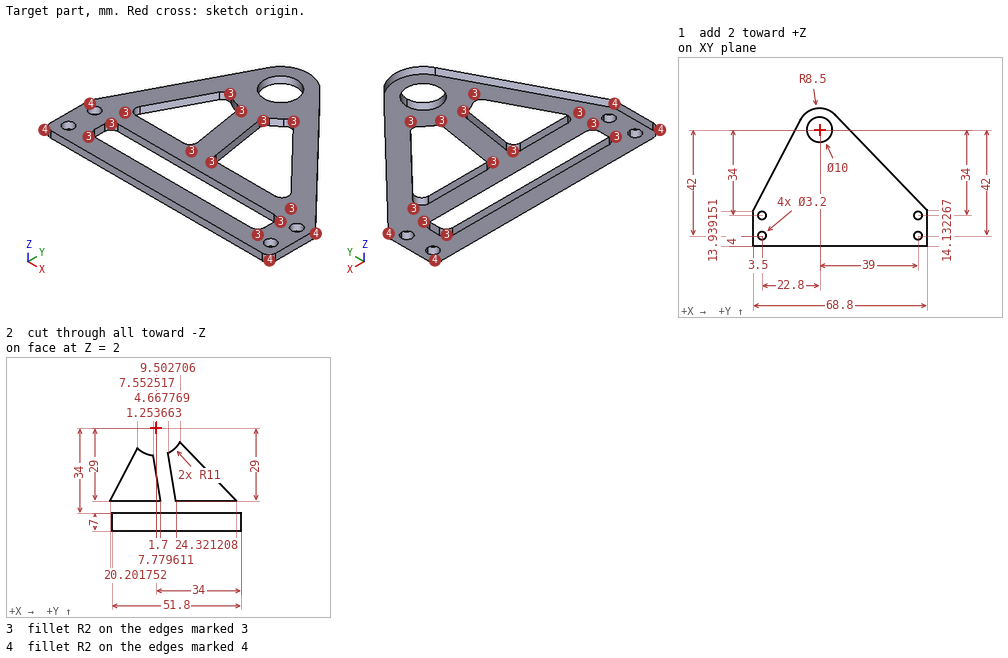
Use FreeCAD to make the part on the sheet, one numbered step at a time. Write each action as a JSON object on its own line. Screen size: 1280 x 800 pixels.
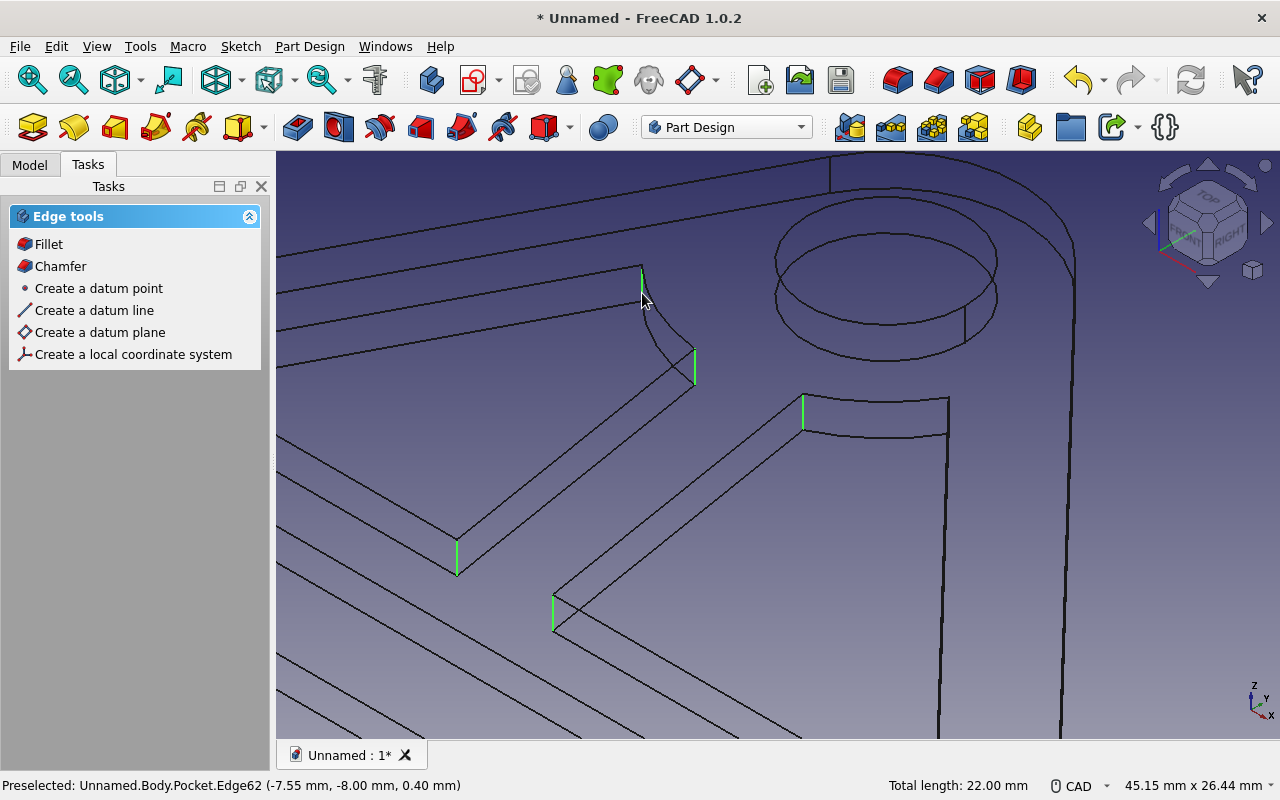
{"action": "left_click", "coordinate": [33, 80]}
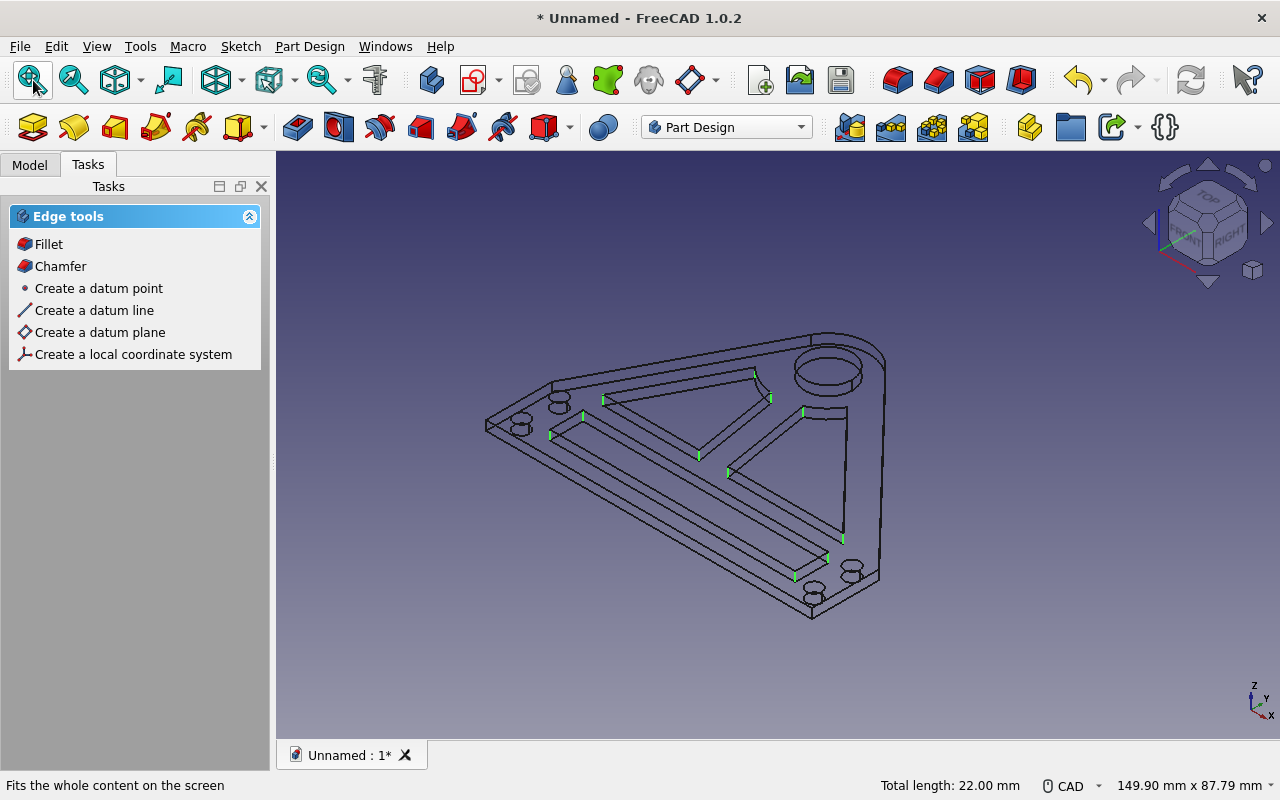
{"action": "key", "text": "2"}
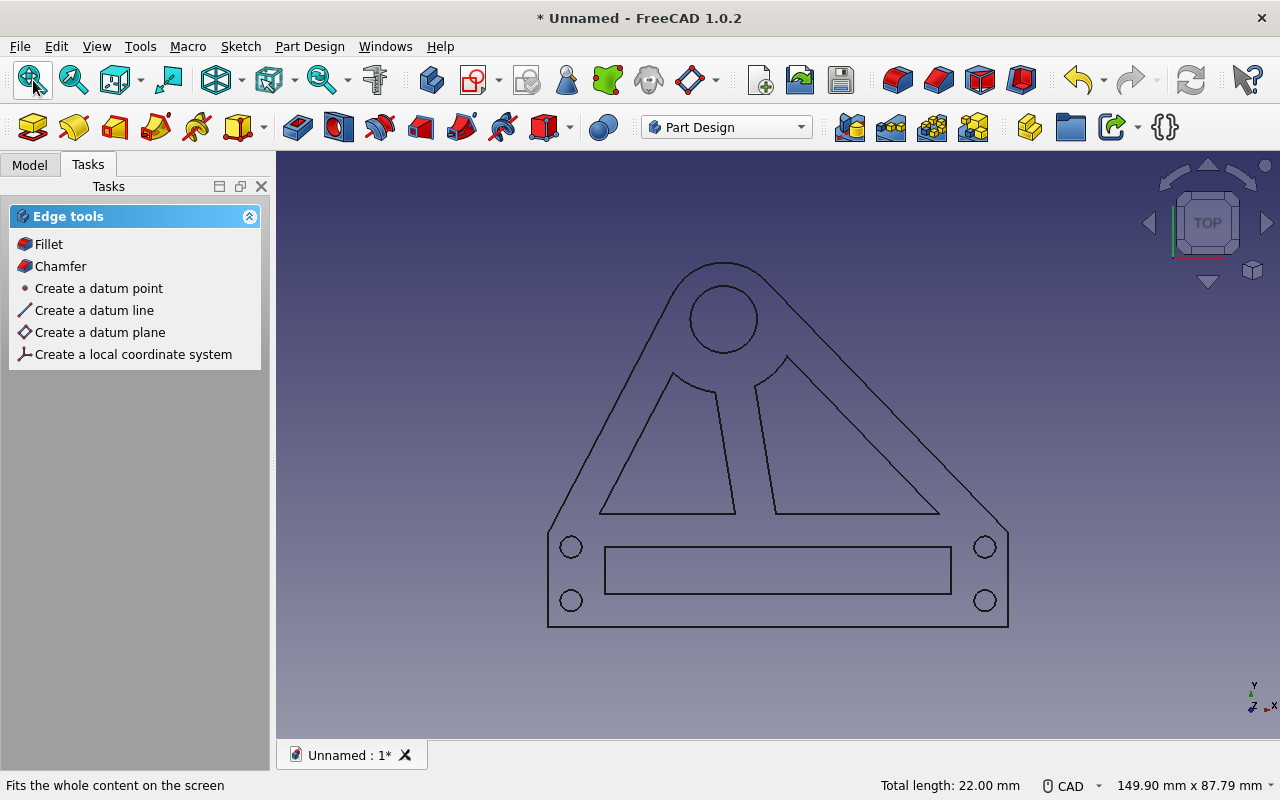
{"action": "scroll", "coordinate": [787, 355], "scroll_direction": "up", "scroll_amount": 6}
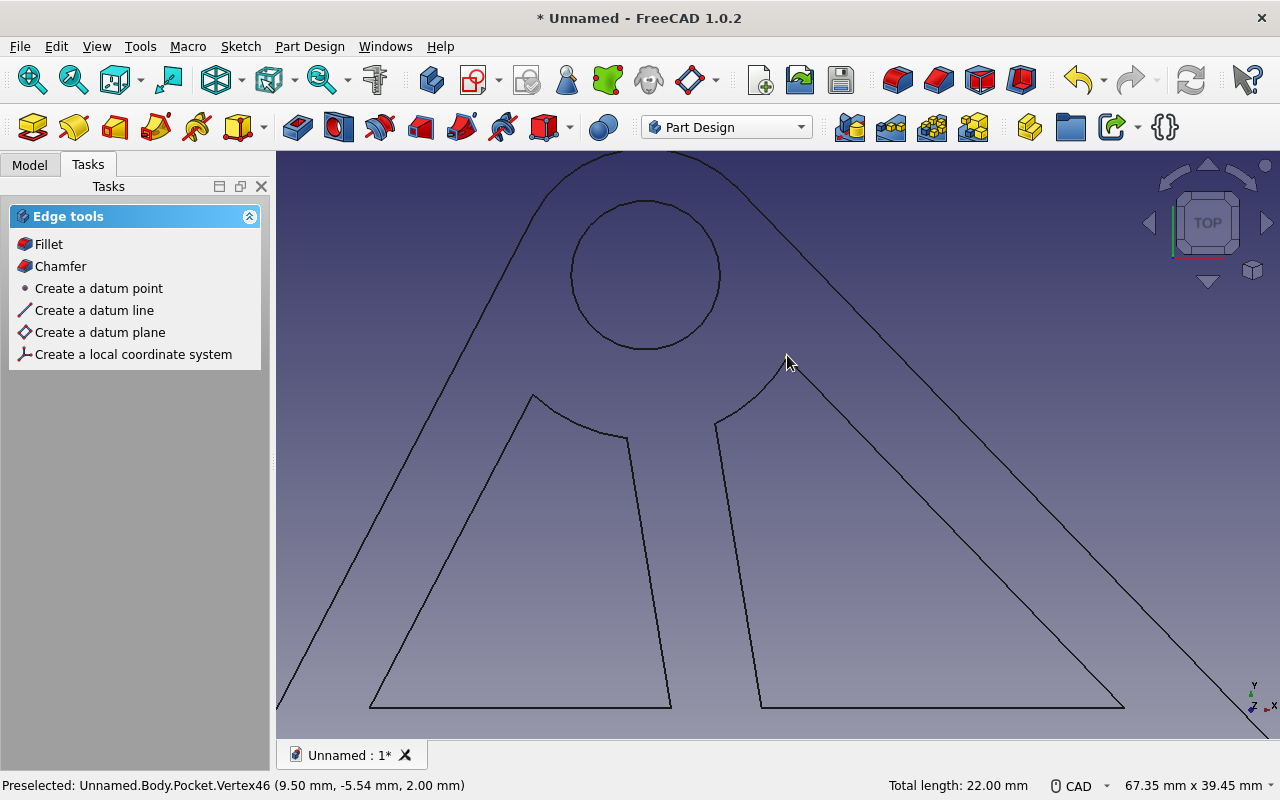
{"action": "left_click", "coordinate": [33, 80]}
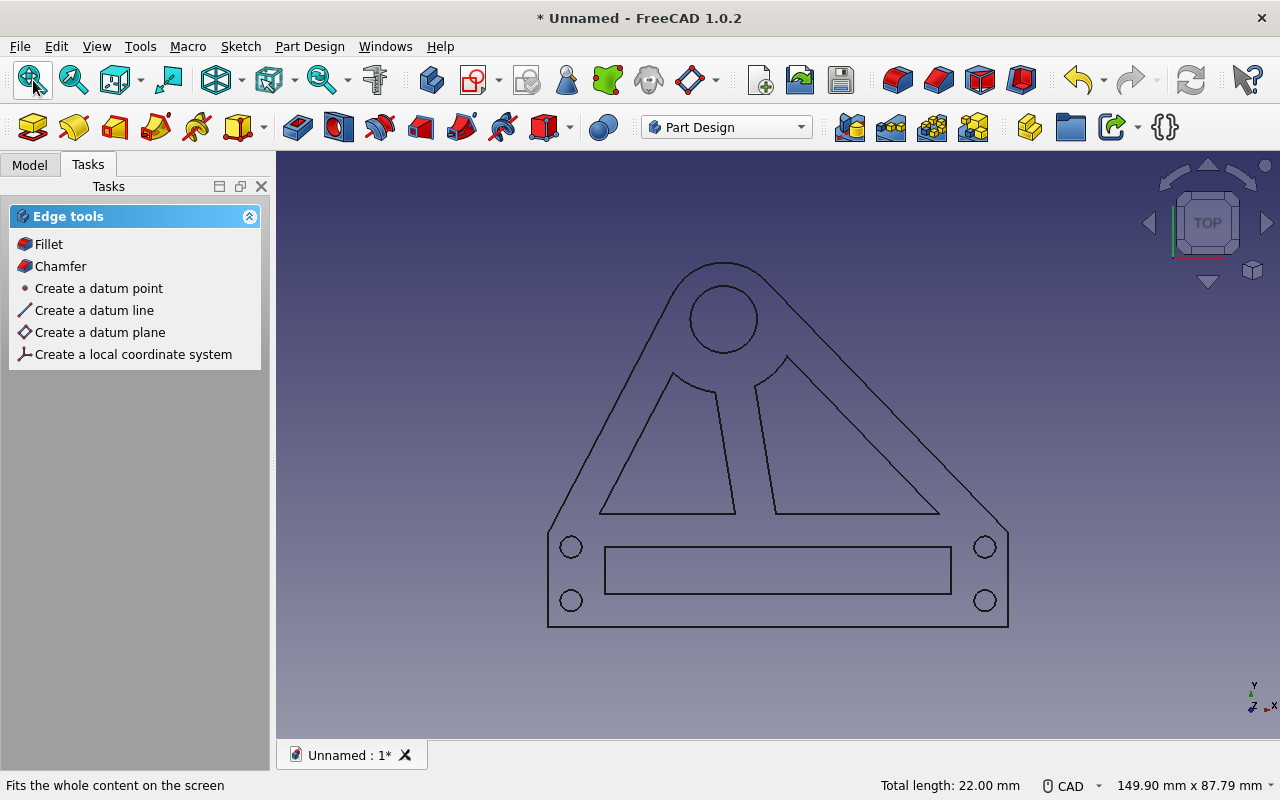
{"action": "key", "text": "1"}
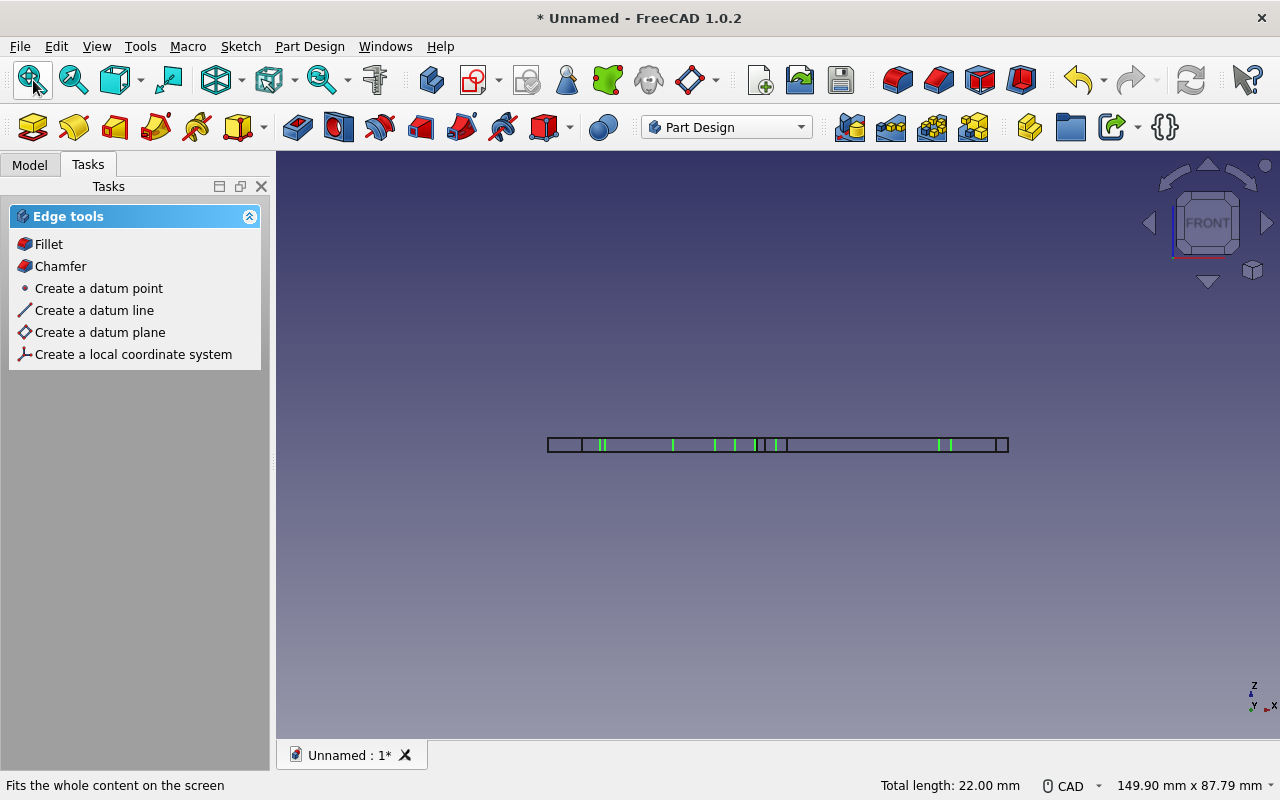
{"action": "left_click", "coordinate": [787, 444], "text": "ctrl"}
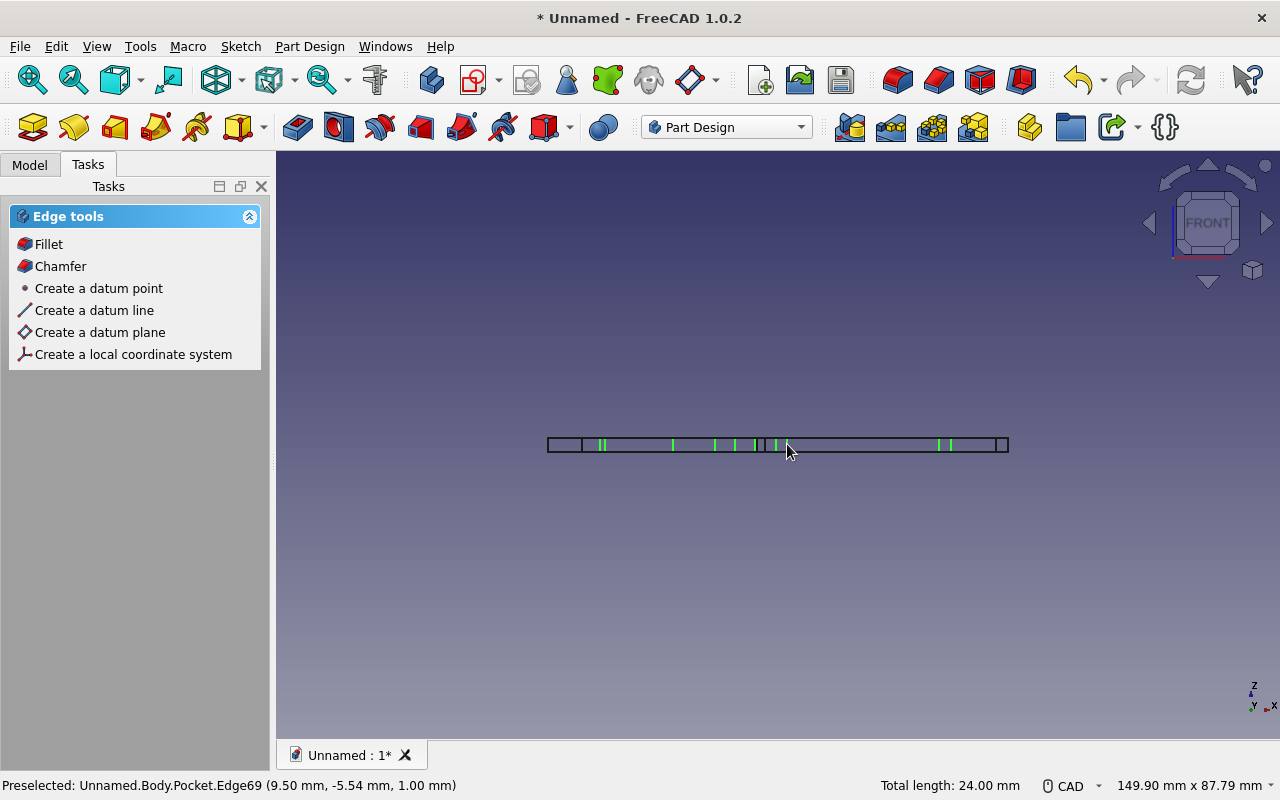
{"action": "key", "text": "v 1"}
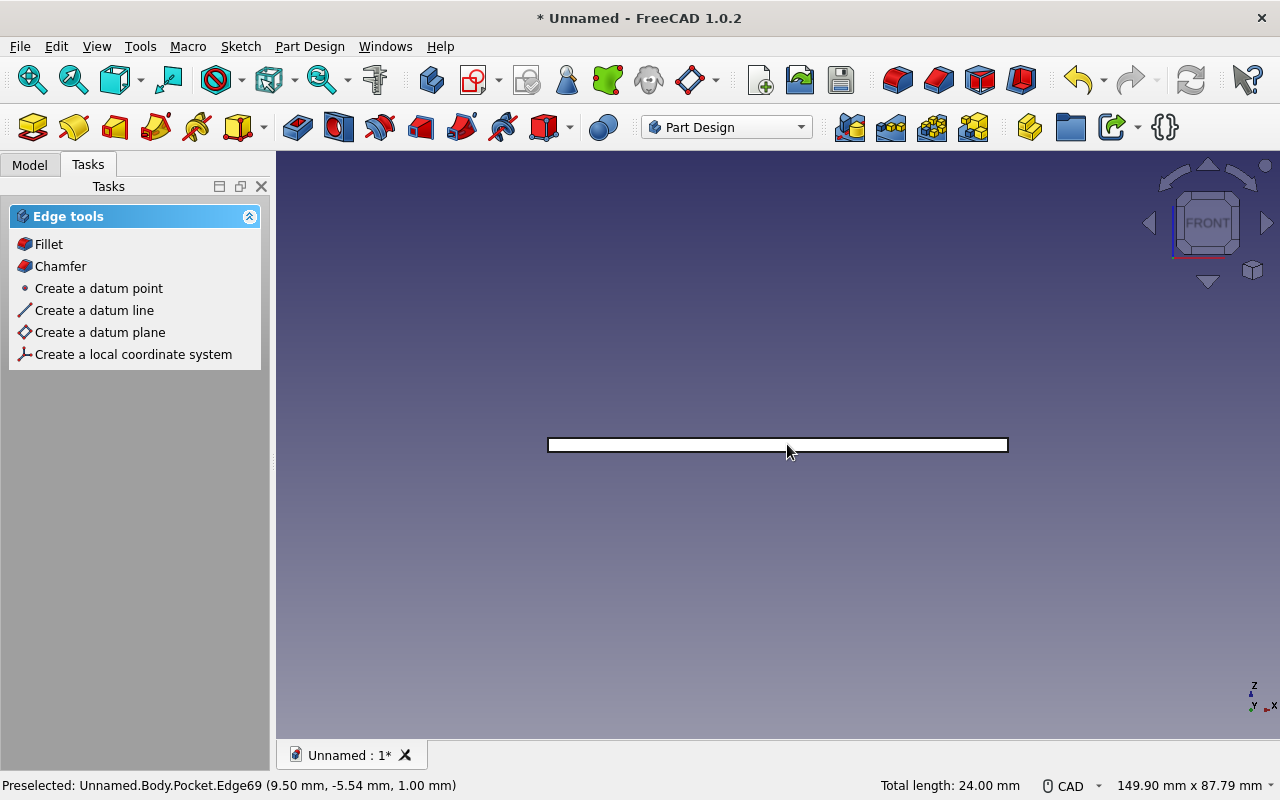
{"action": "left_click", "coordinate": [898, 80]}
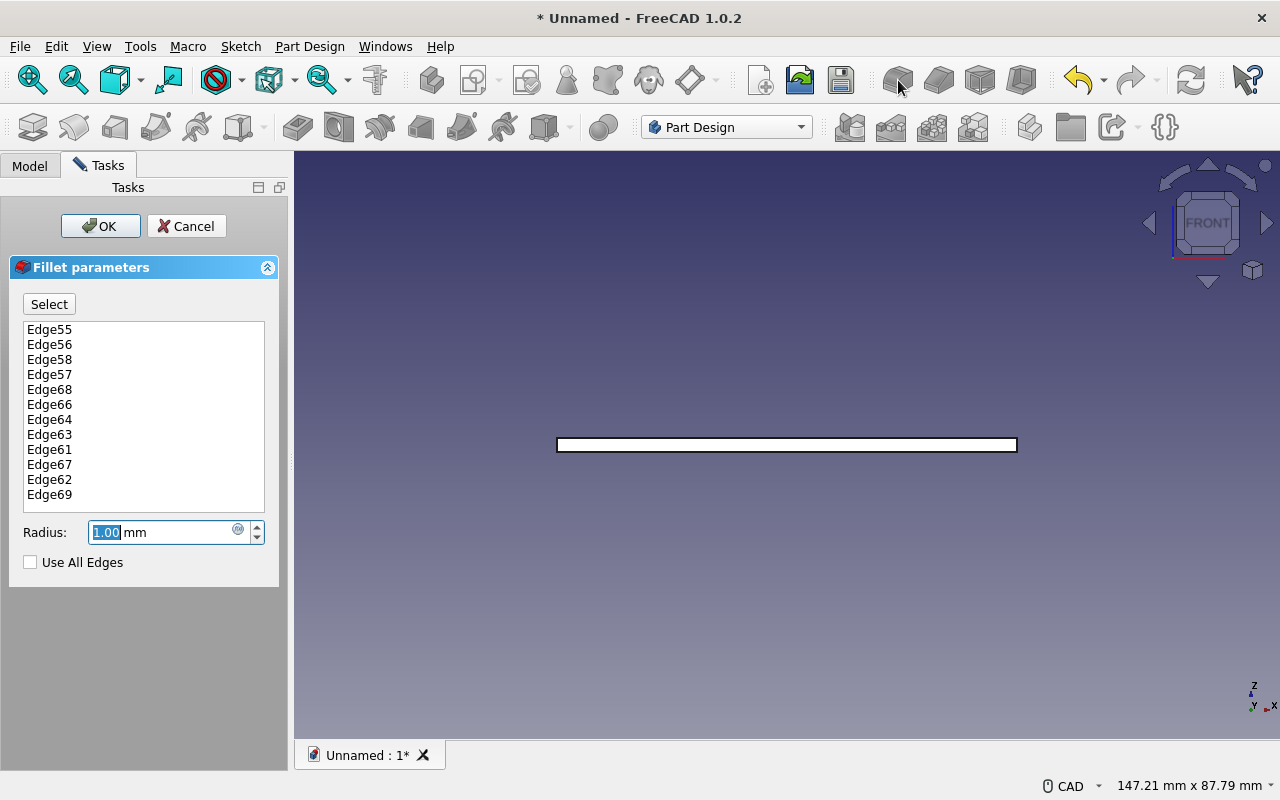
{"action": "type", "text": "2"}
{"action": "key", "text": "Tab"}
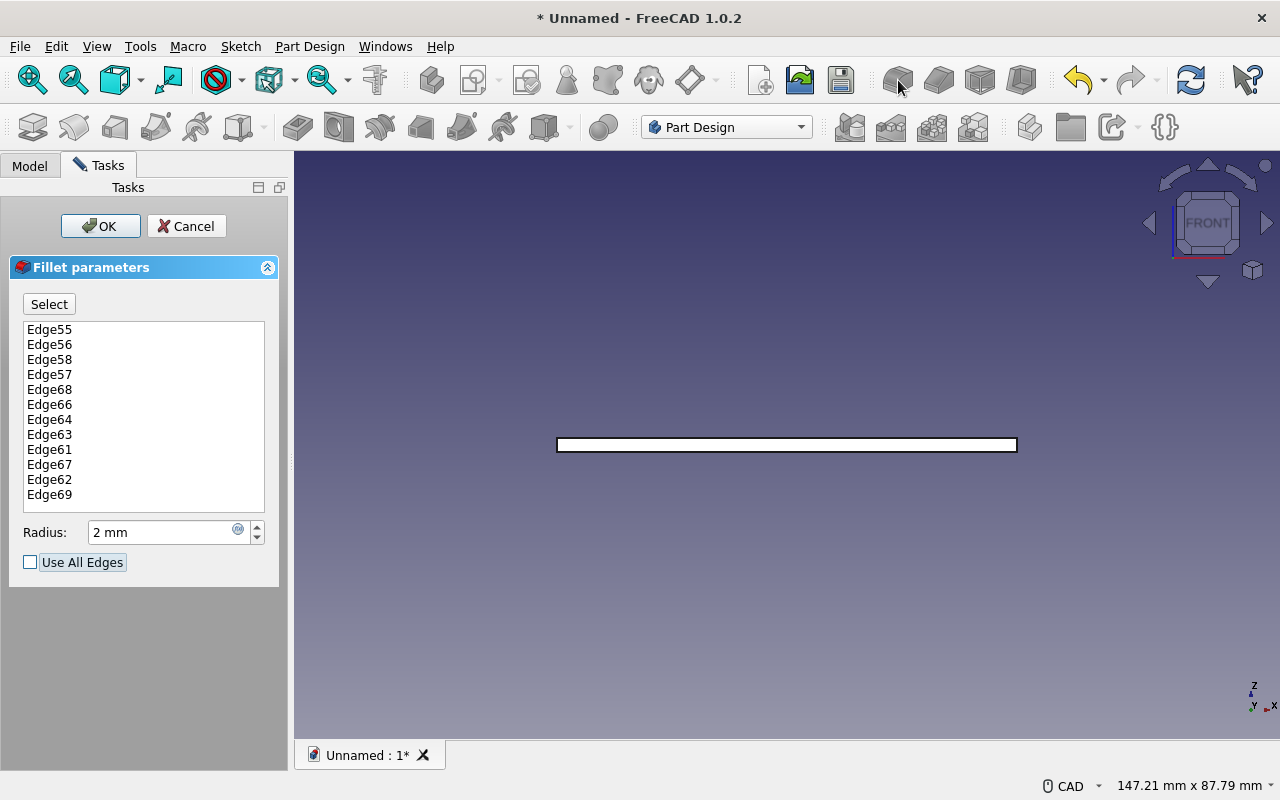
{"action": "left_click", "coordinate": [101, 226]}